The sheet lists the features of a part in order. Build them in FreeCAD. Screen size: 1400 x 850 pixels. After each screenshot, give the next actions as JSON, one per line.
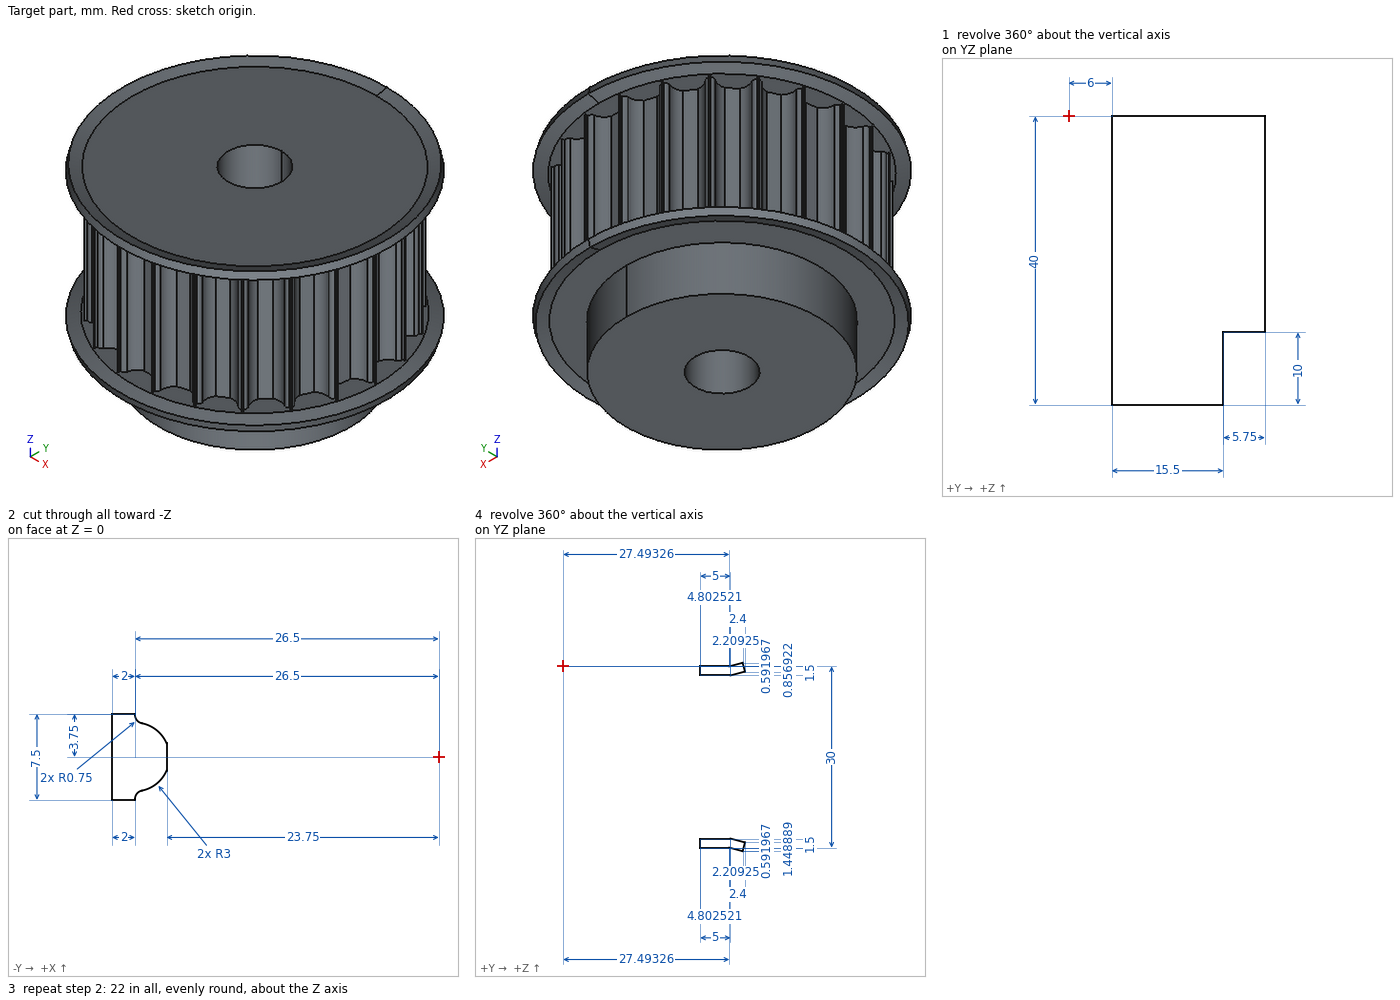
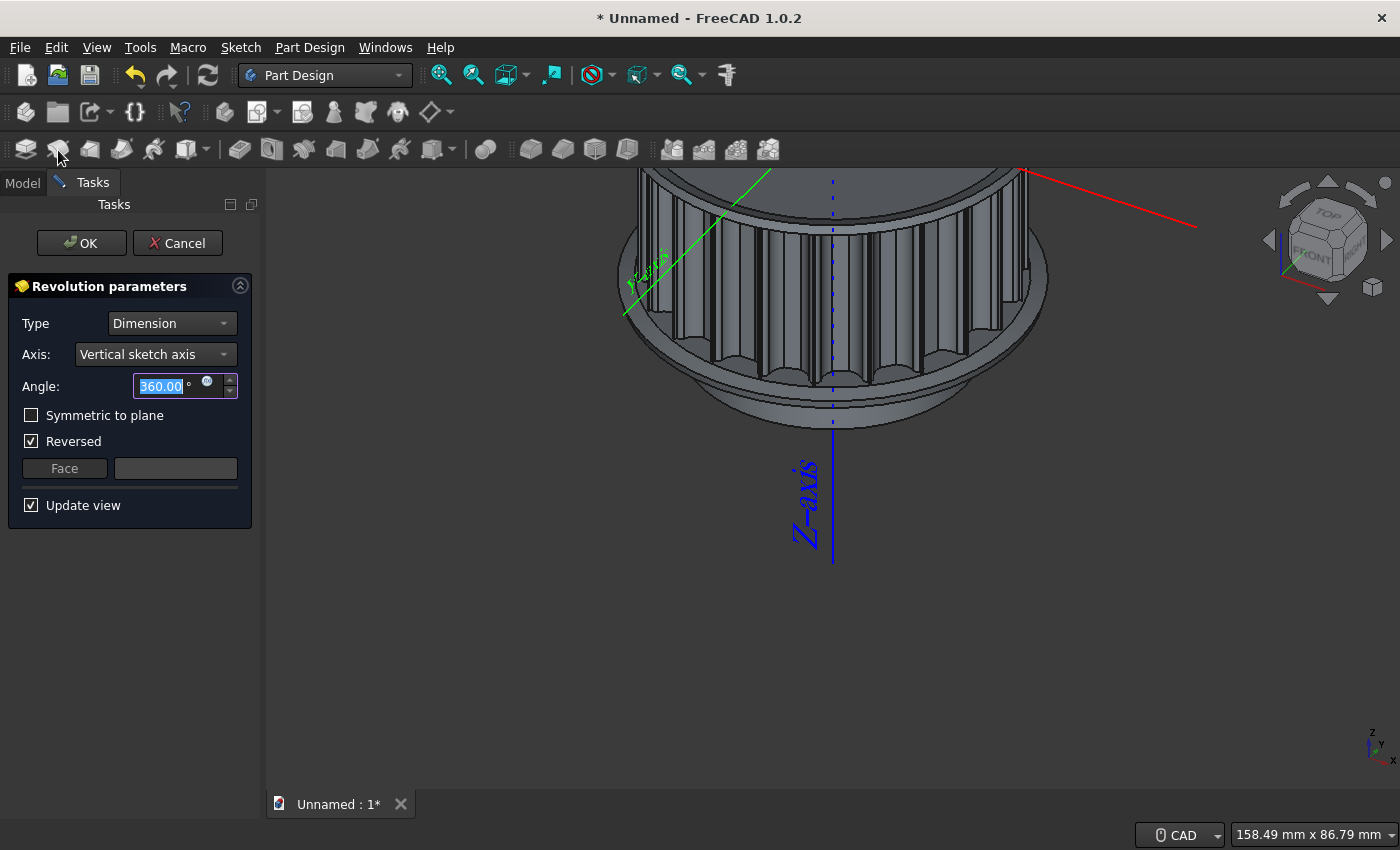
{"action": "left_click", "coordinate": [82, 243]}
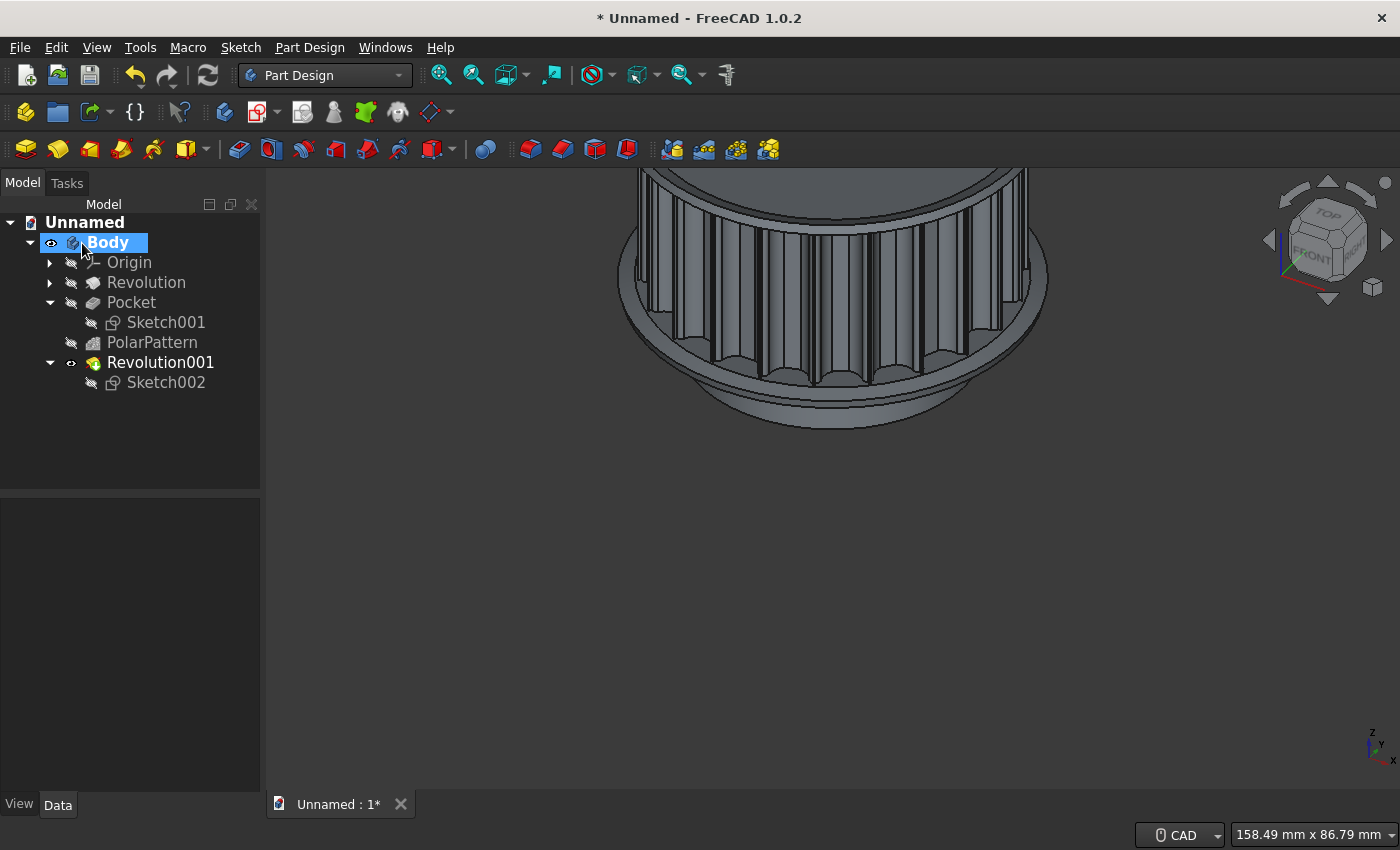
{"action": "key", "text": "0"}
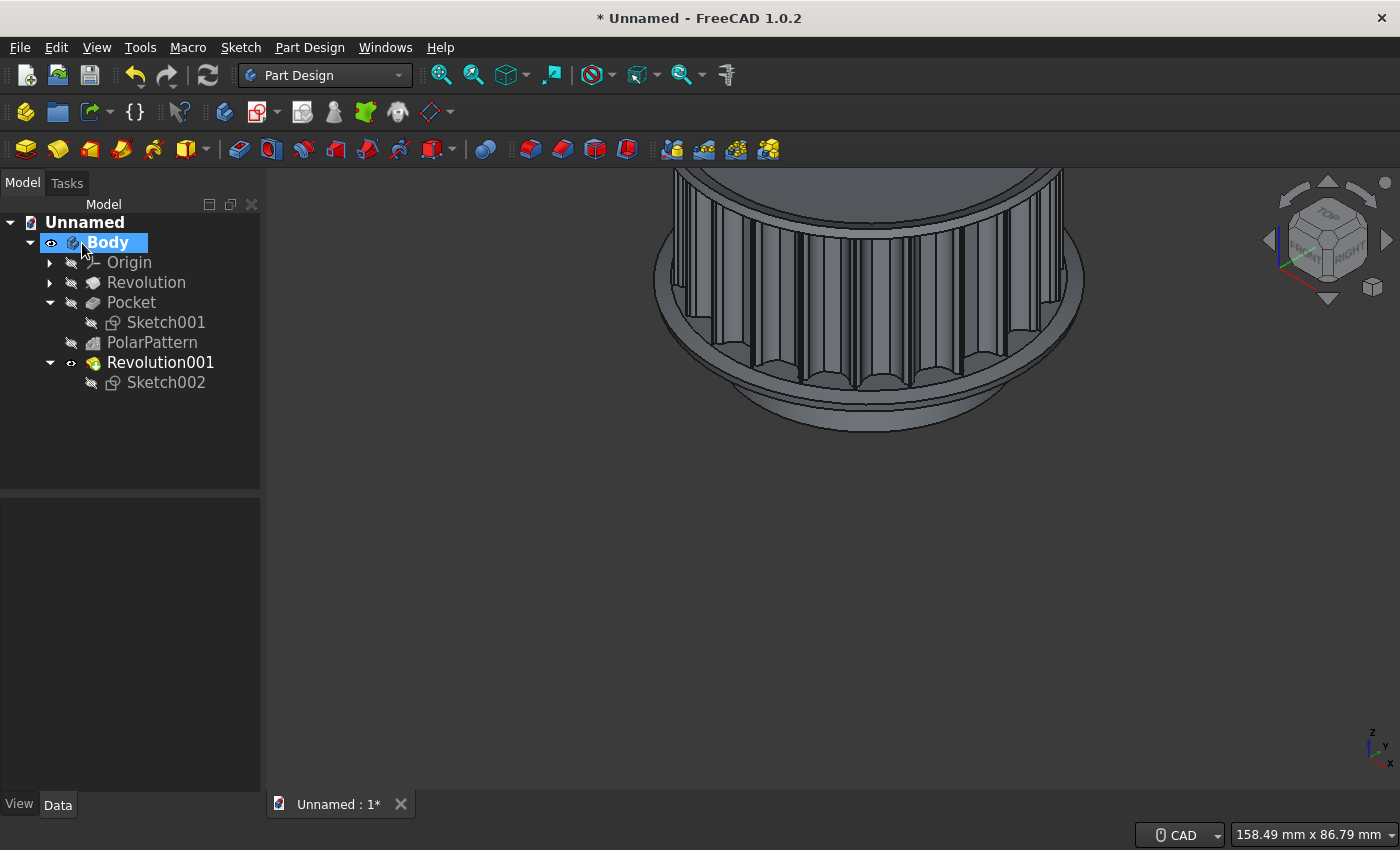
{"action": "key", "text": "v f"}